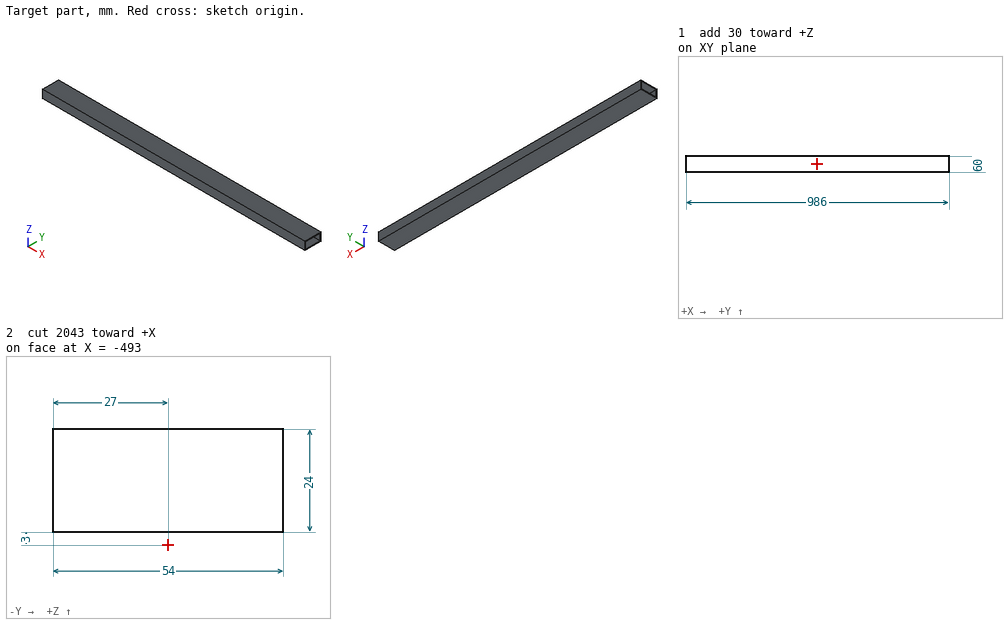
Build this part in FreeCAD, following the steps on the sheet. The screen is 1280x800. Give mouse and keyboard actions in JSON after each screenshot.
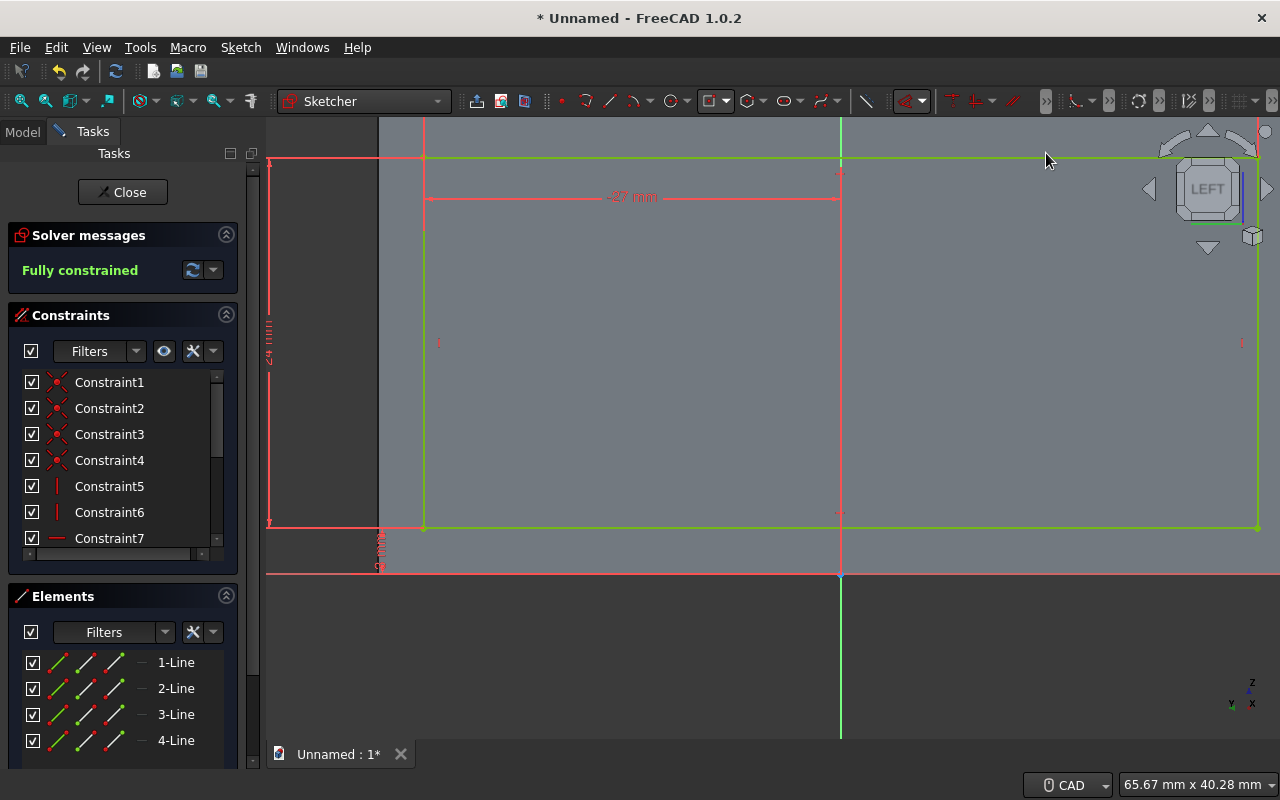
{"action": "left_click", "coordinate": [123, 192]}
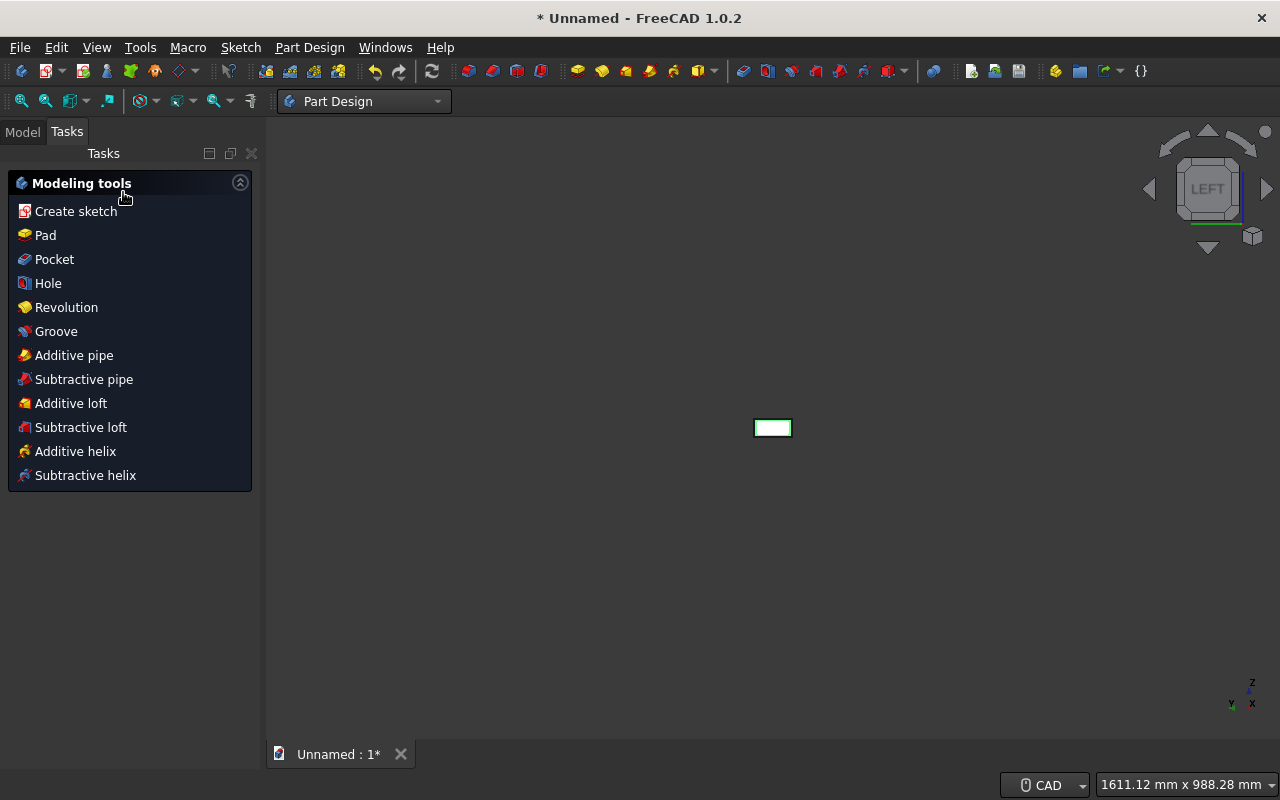
{"action": "left_click", "coordinate": [744, 72]}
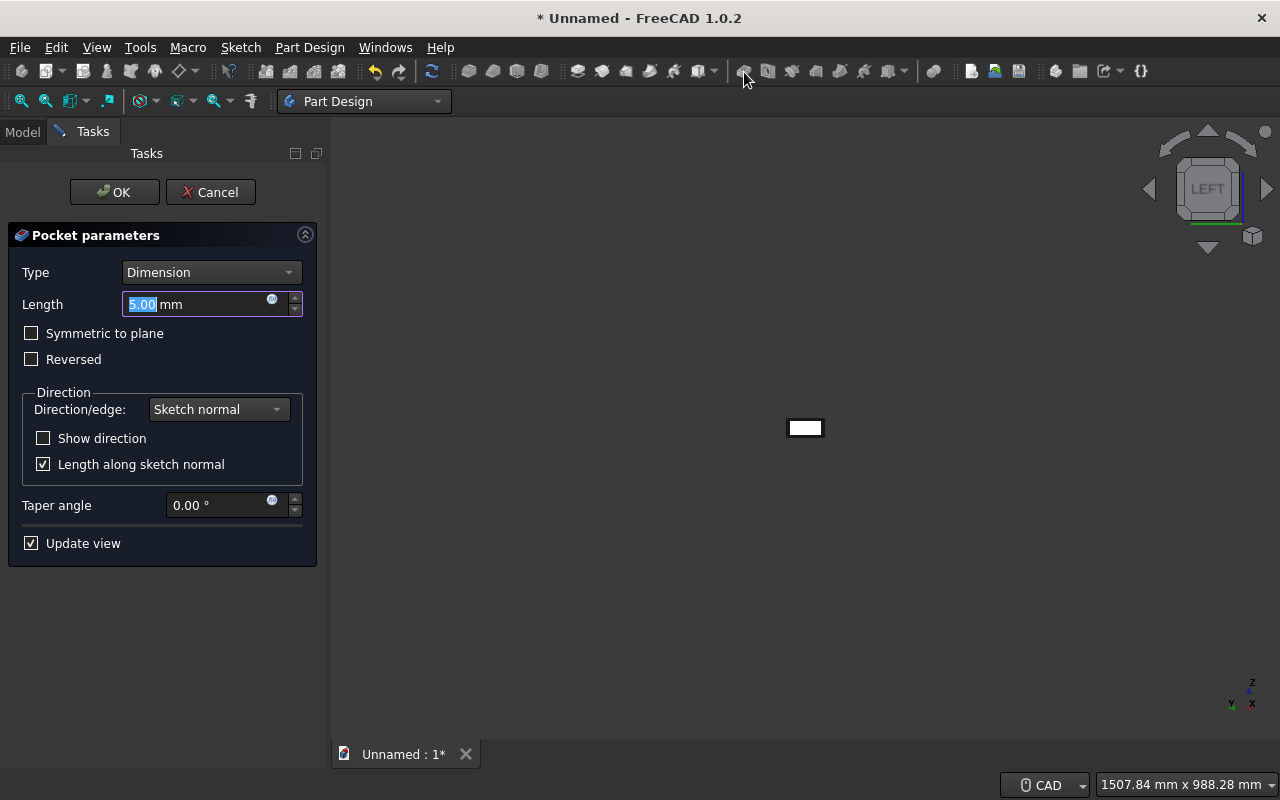
{"action": "type", "text": "2043"}
{"action": "key", "text": "Tab"}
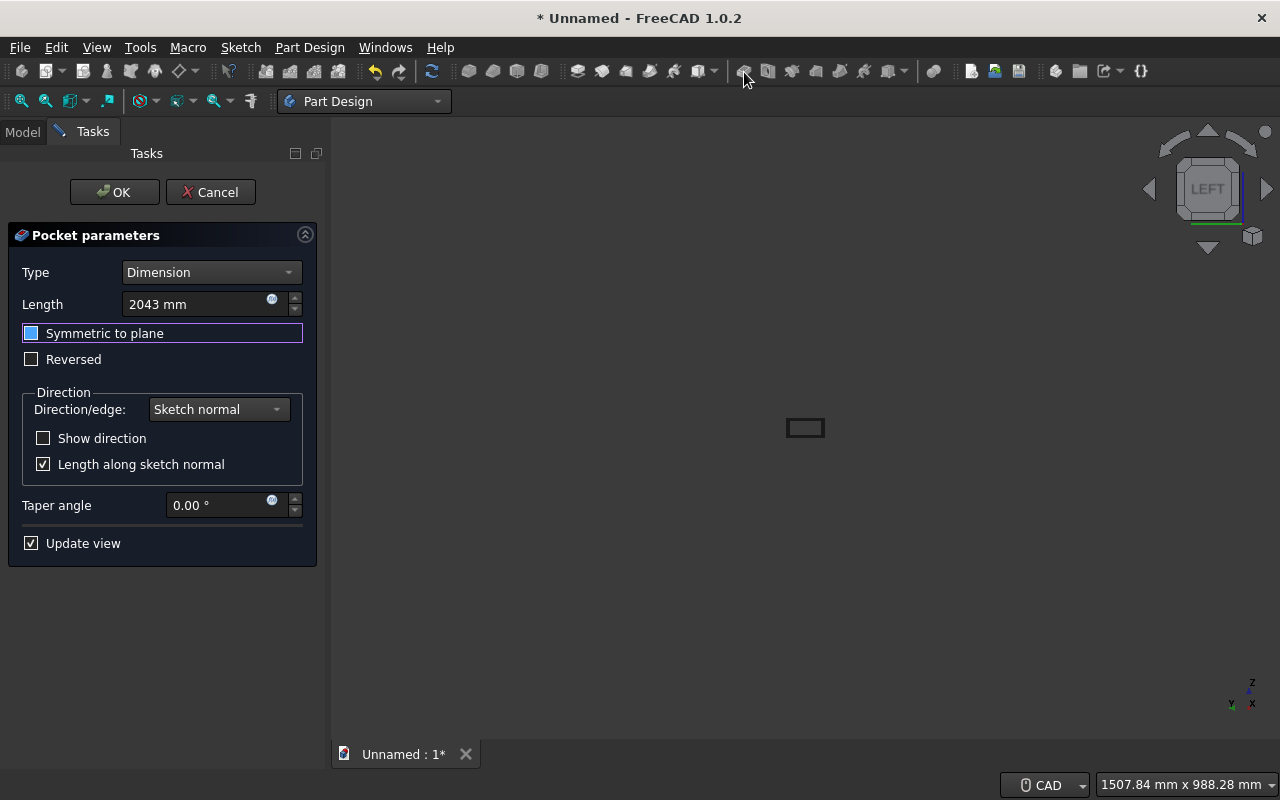
{"action": "left_click", "coordinate": [115, 192]}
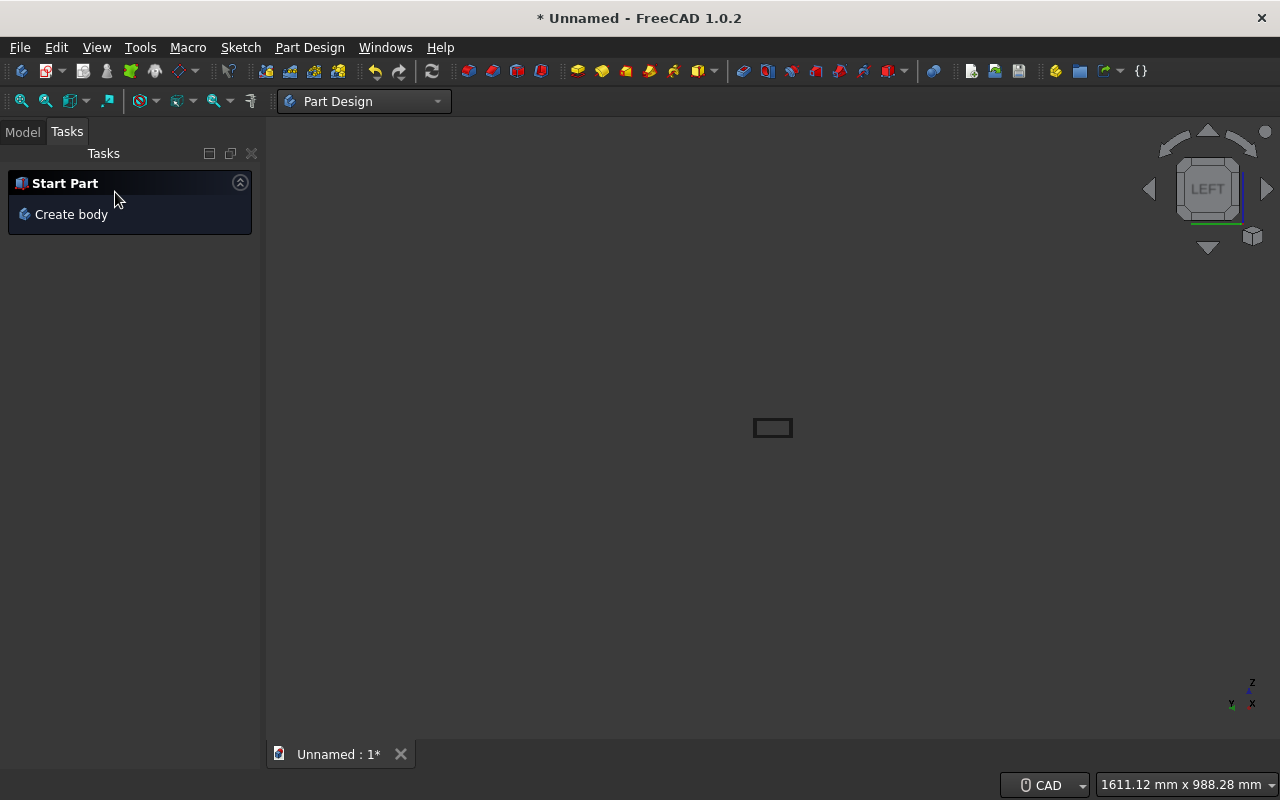
{"action": "key", "text": "0"}